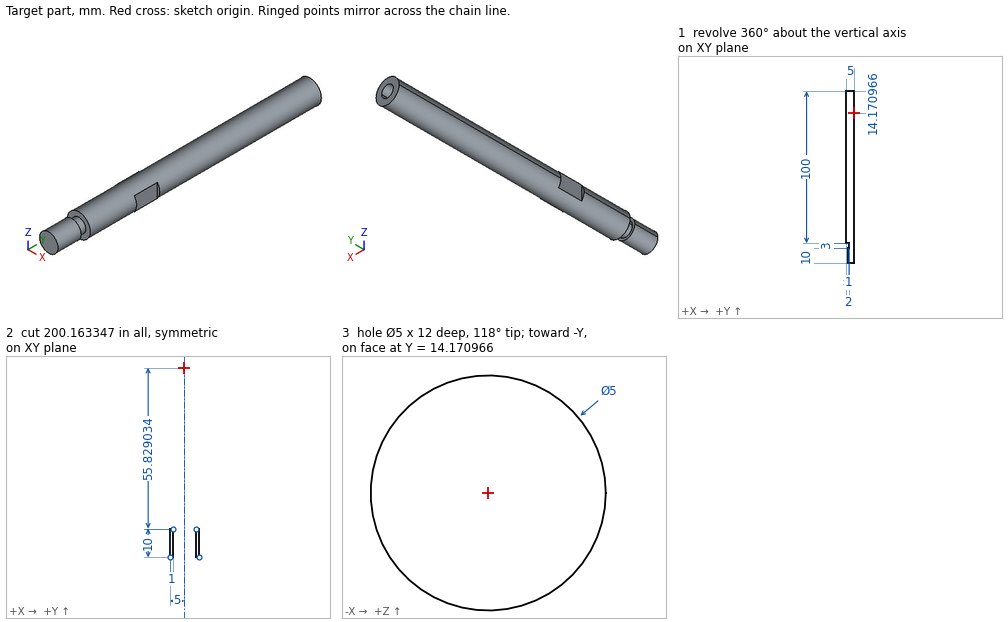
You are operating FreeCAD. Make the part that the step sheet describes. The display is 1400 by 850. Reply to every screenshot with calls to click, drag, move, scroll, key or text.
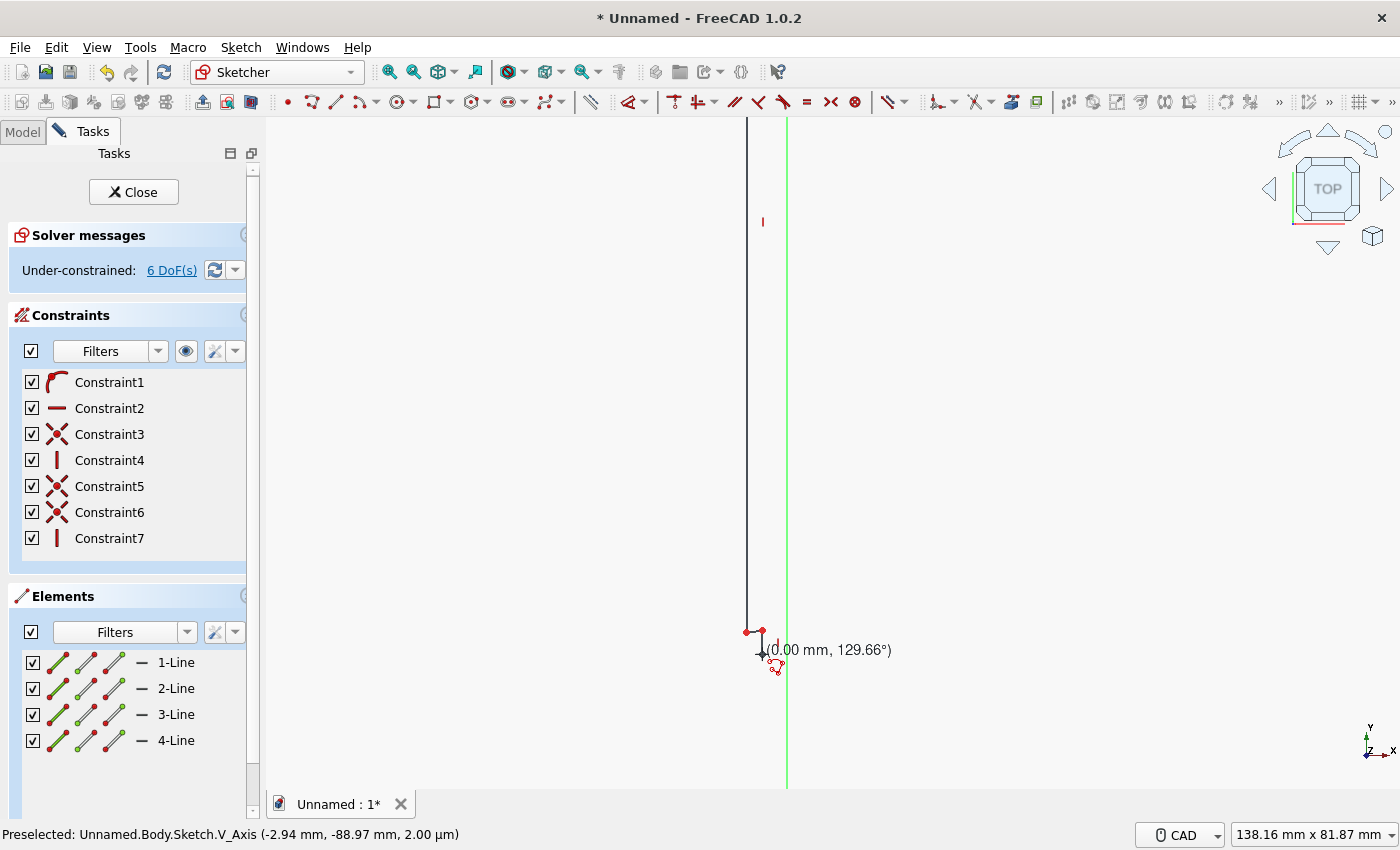
scroll(754, 654, up, 4)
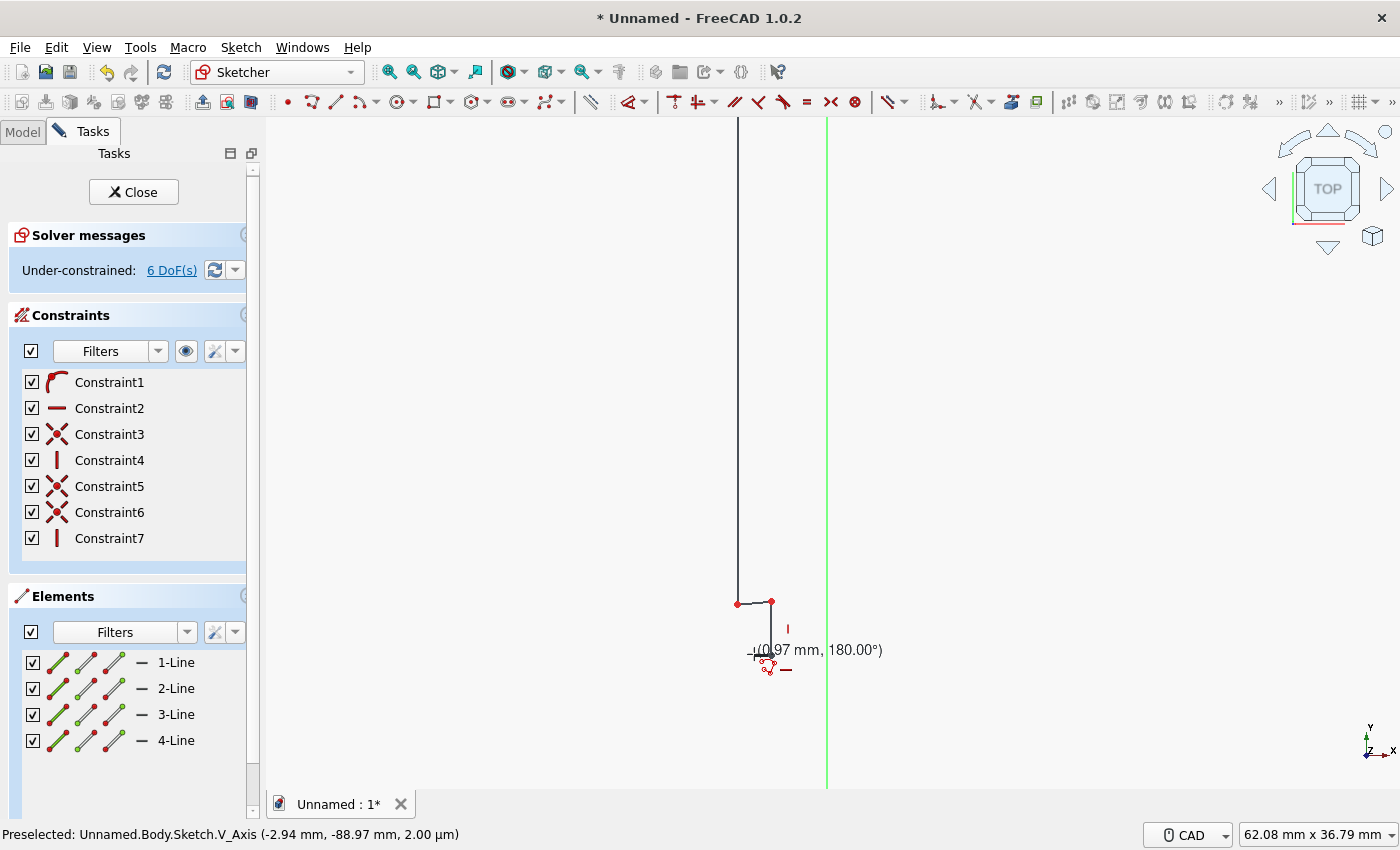
click(754, 653)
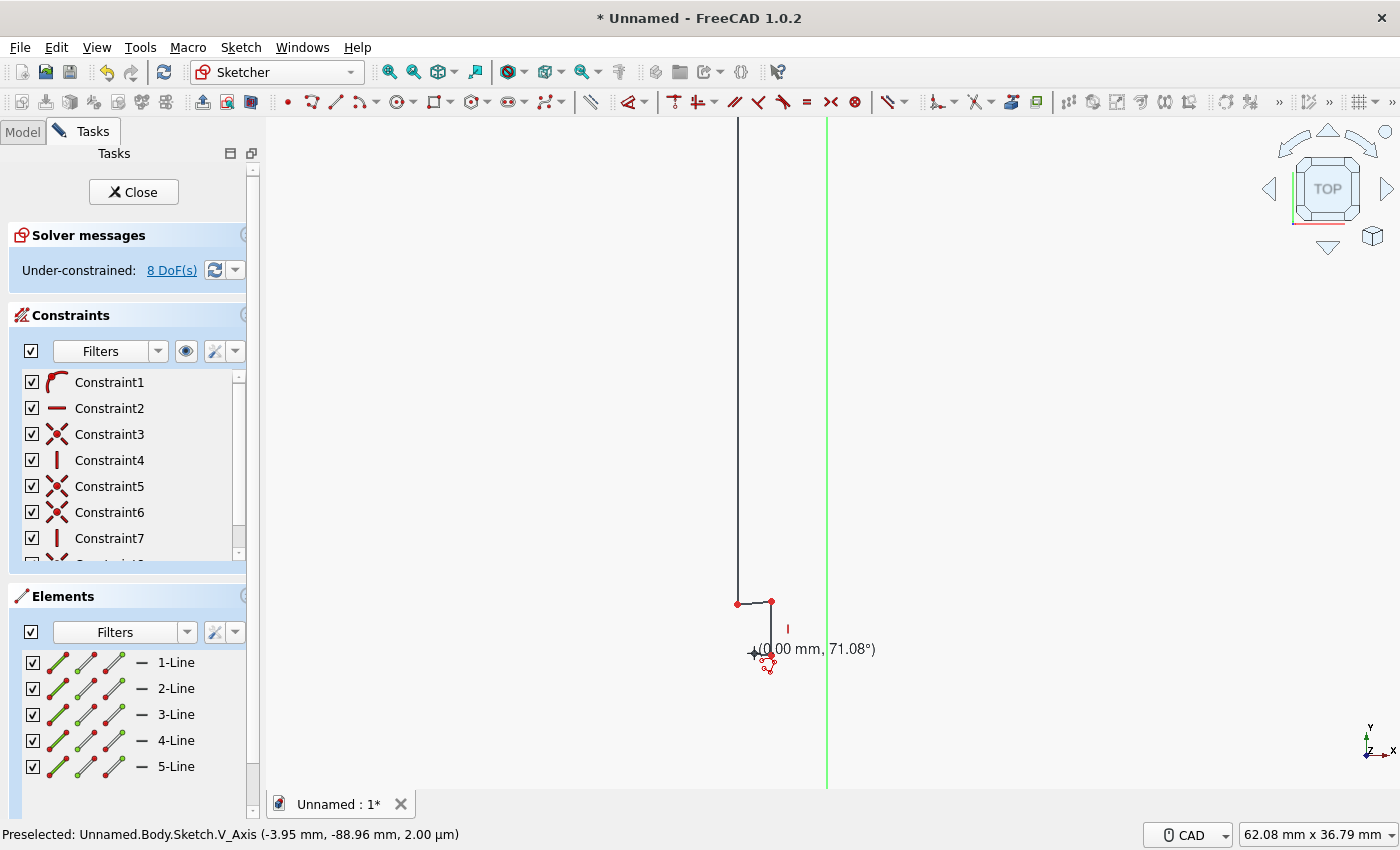
scroll(760, 617, down, 8)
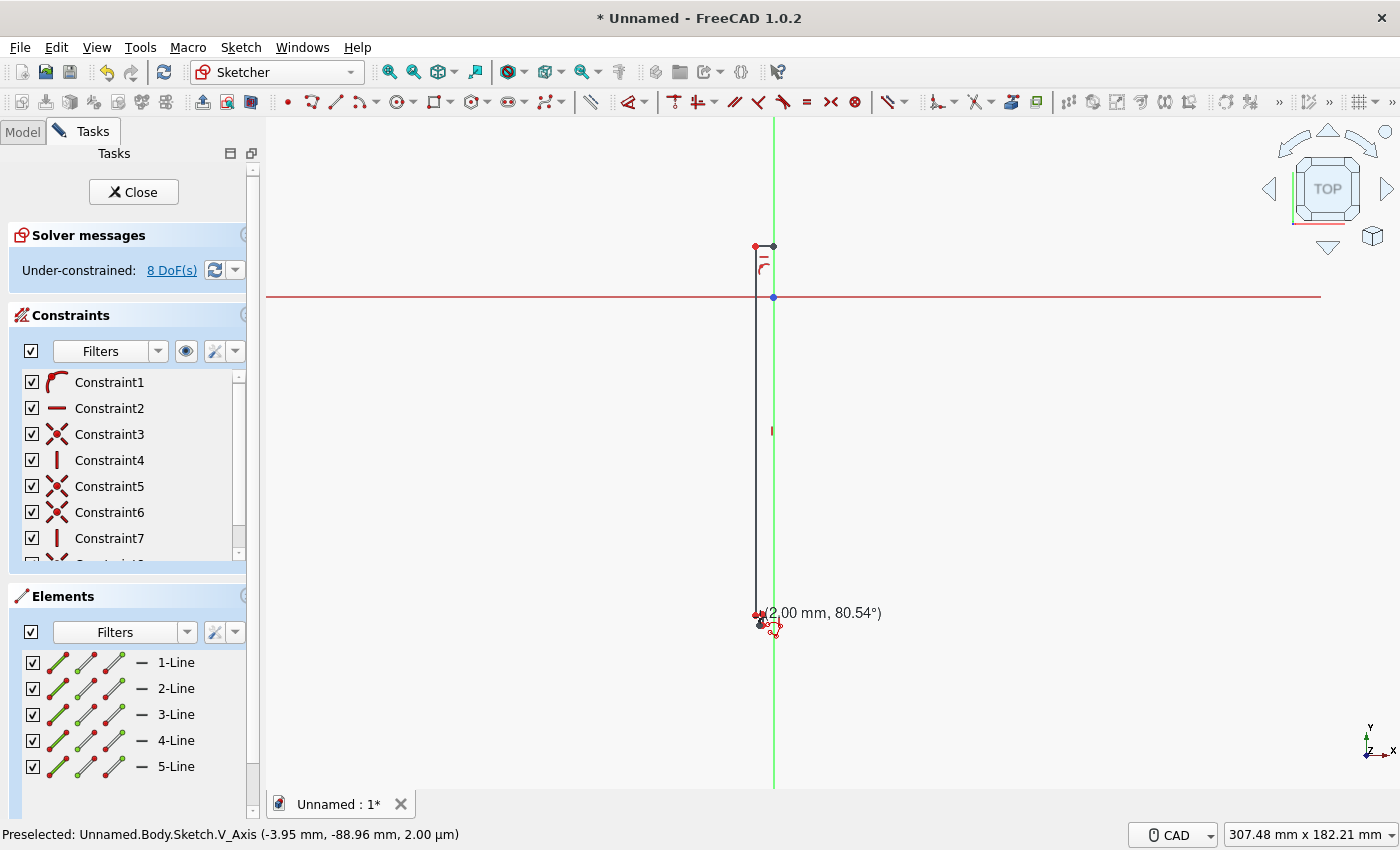
click(759, 662)
click(765, 662)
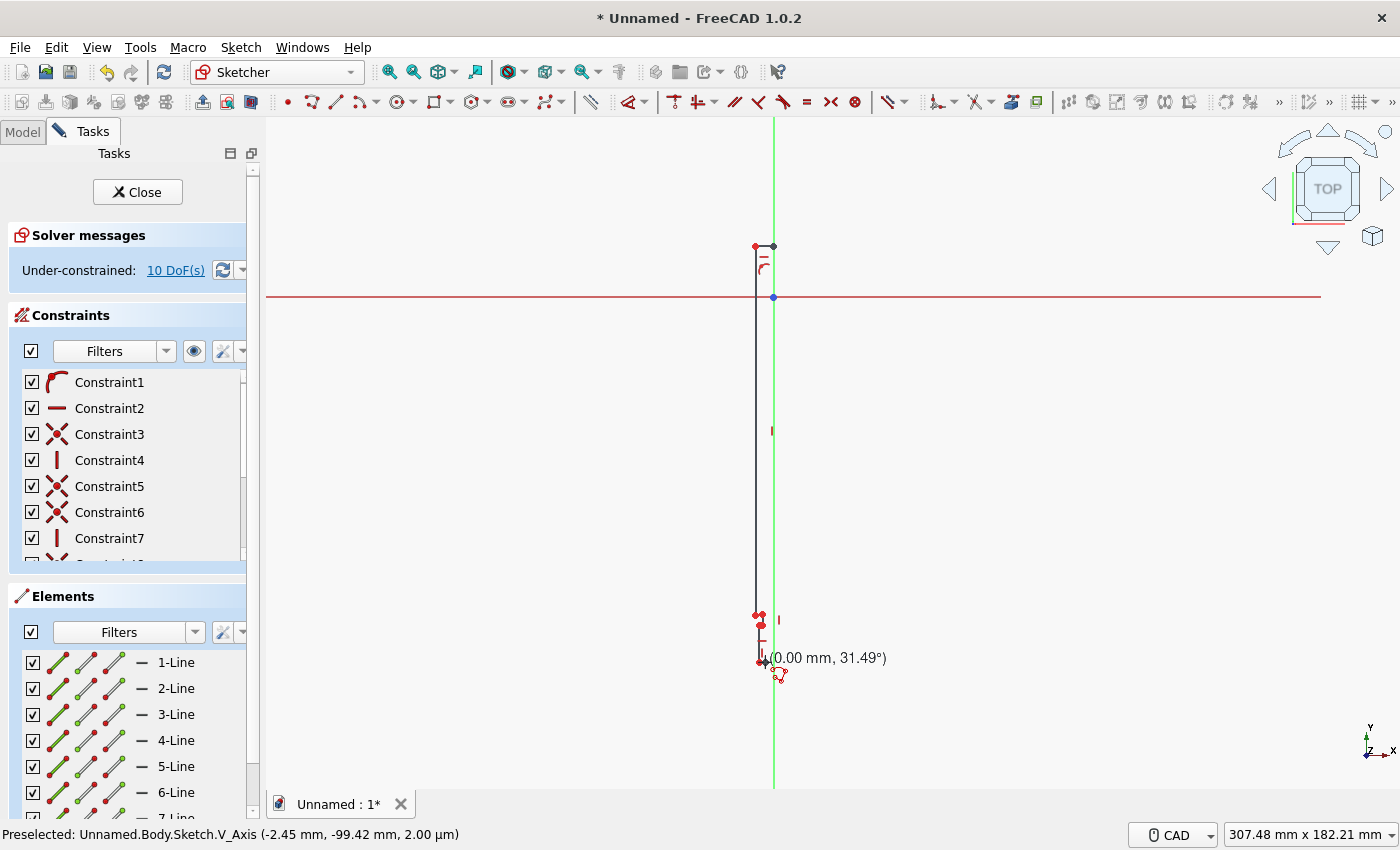
scroll(774, 245, up, 3)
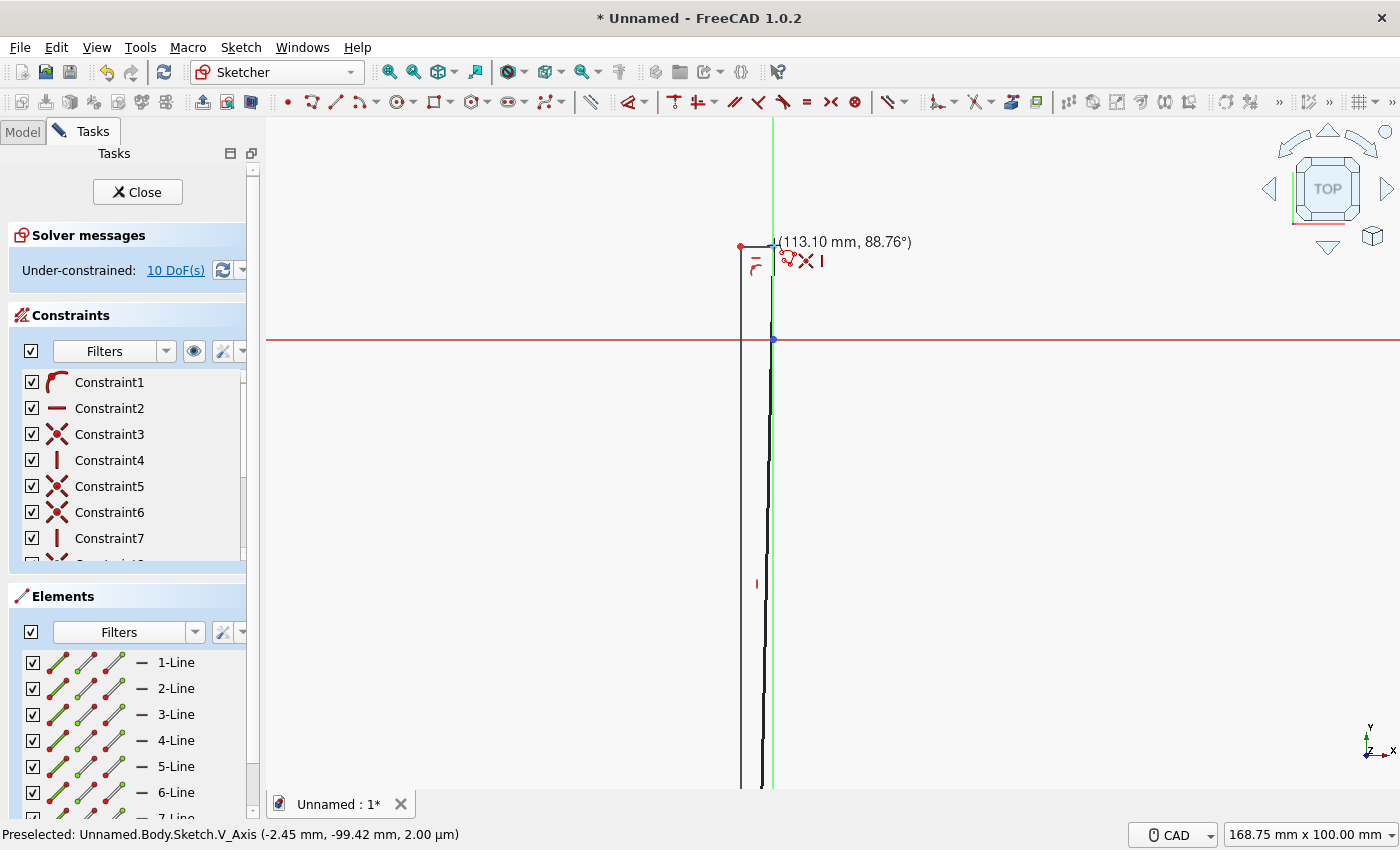
click(773, 247)
key(Escape)
key(Escape)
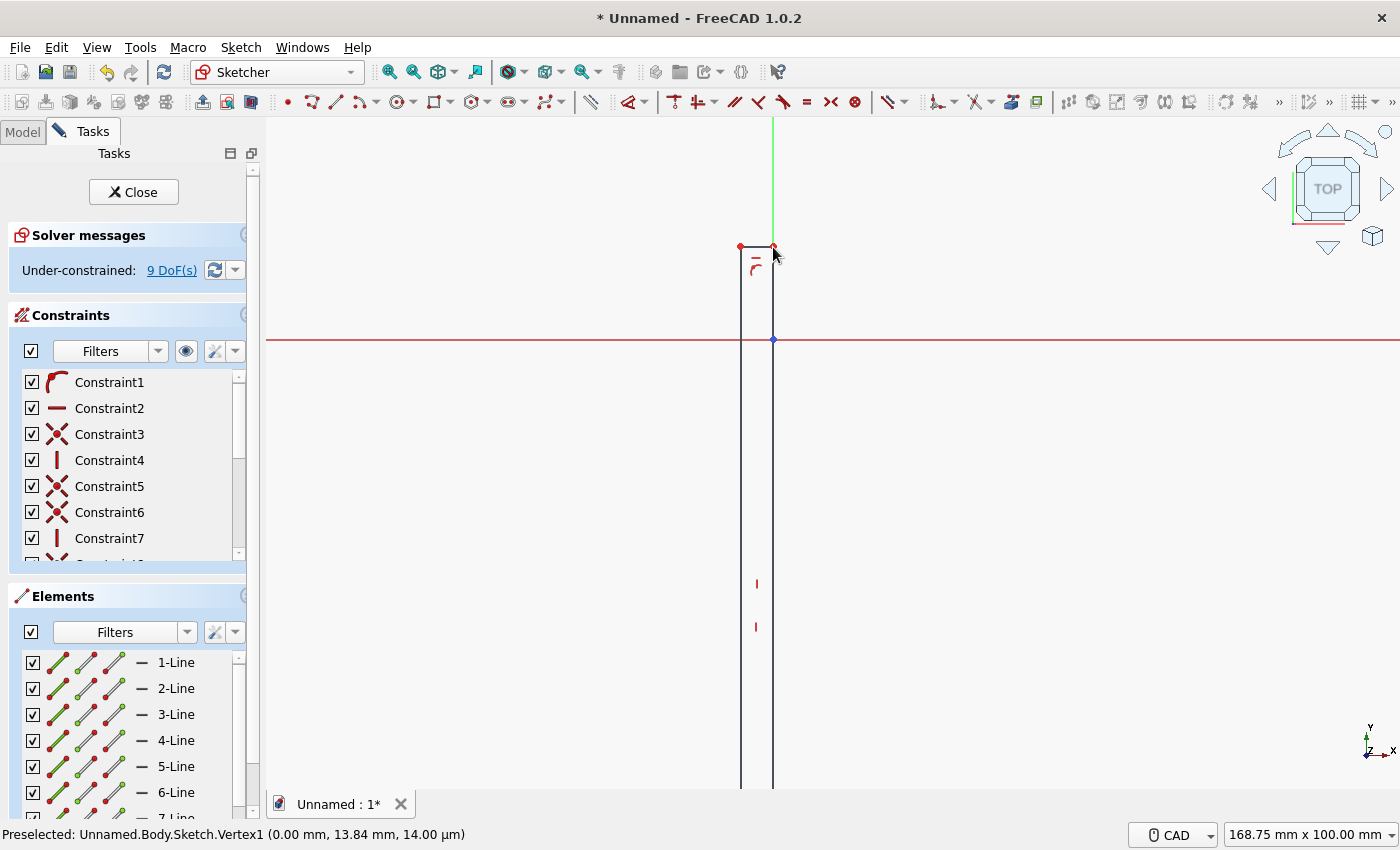
scroll(774, 245, down, 3)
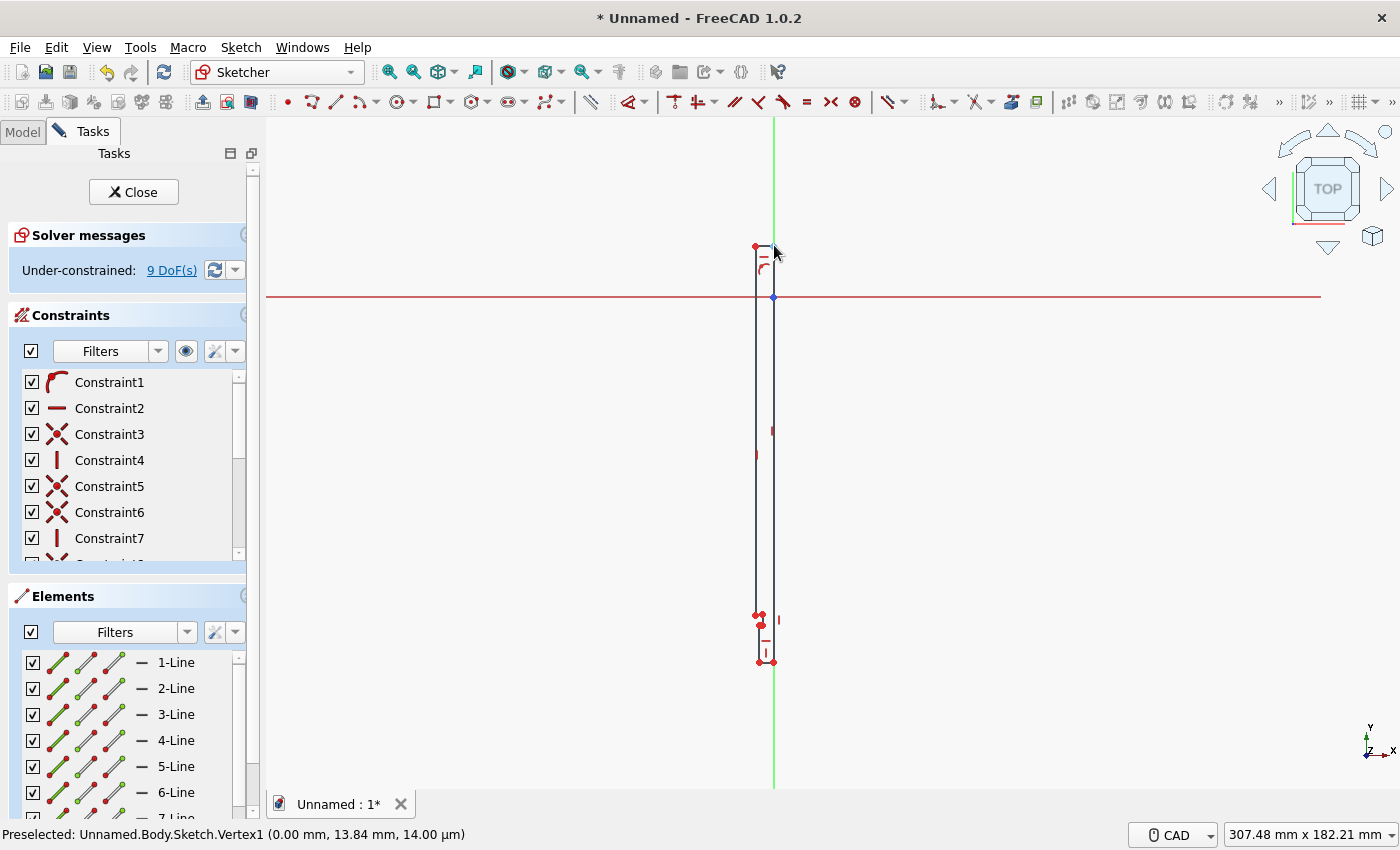
scroll(759, 615, up, 8)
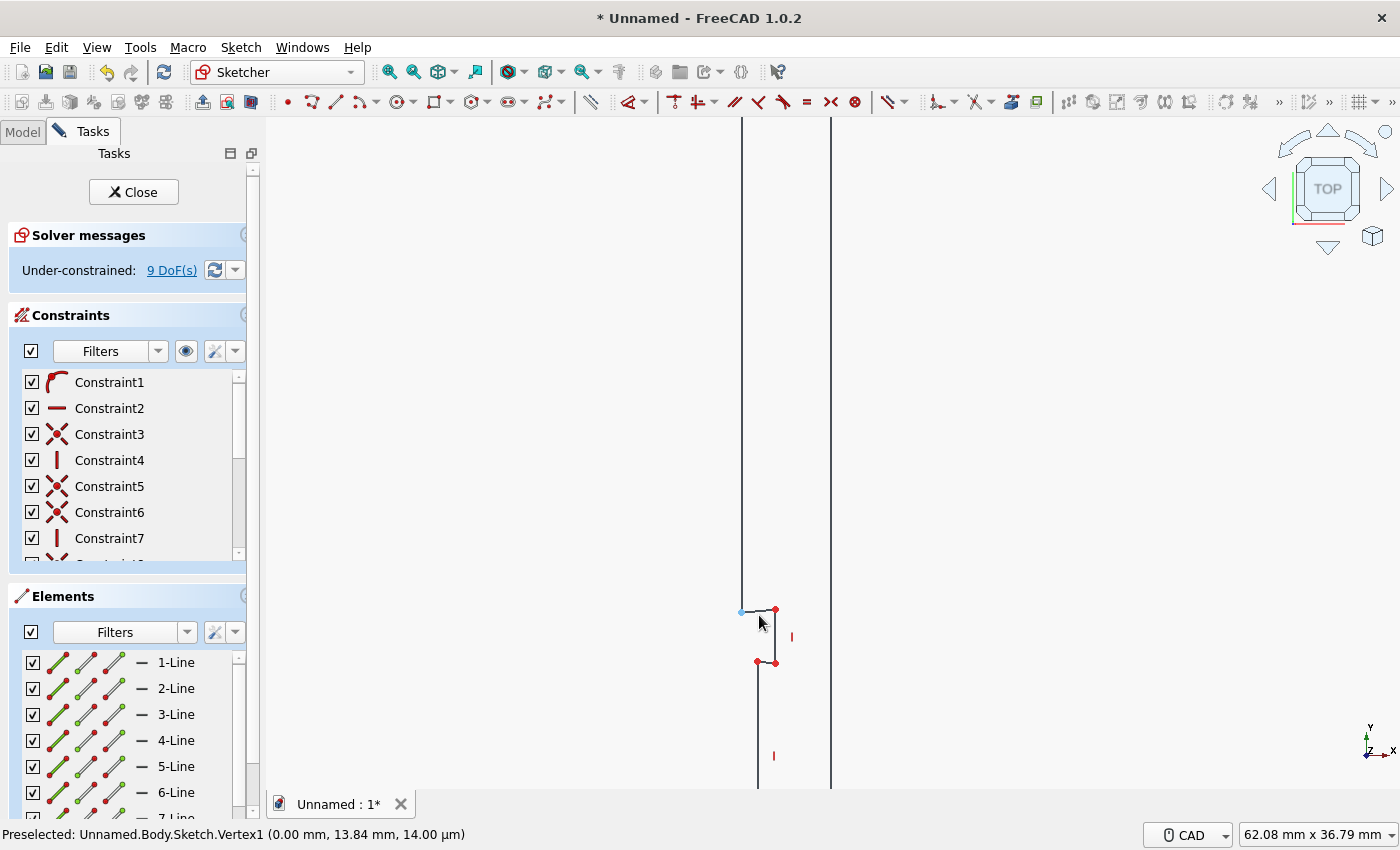
click(758, 611)